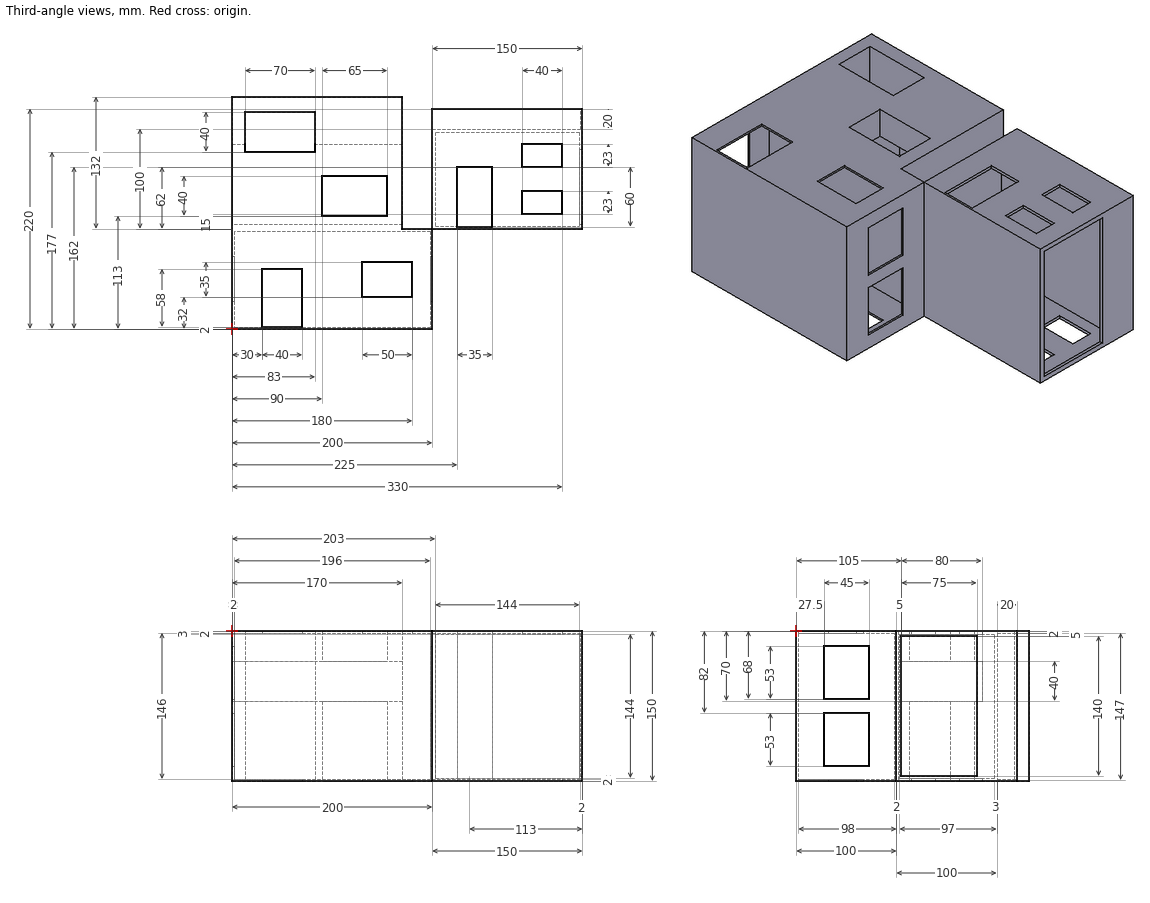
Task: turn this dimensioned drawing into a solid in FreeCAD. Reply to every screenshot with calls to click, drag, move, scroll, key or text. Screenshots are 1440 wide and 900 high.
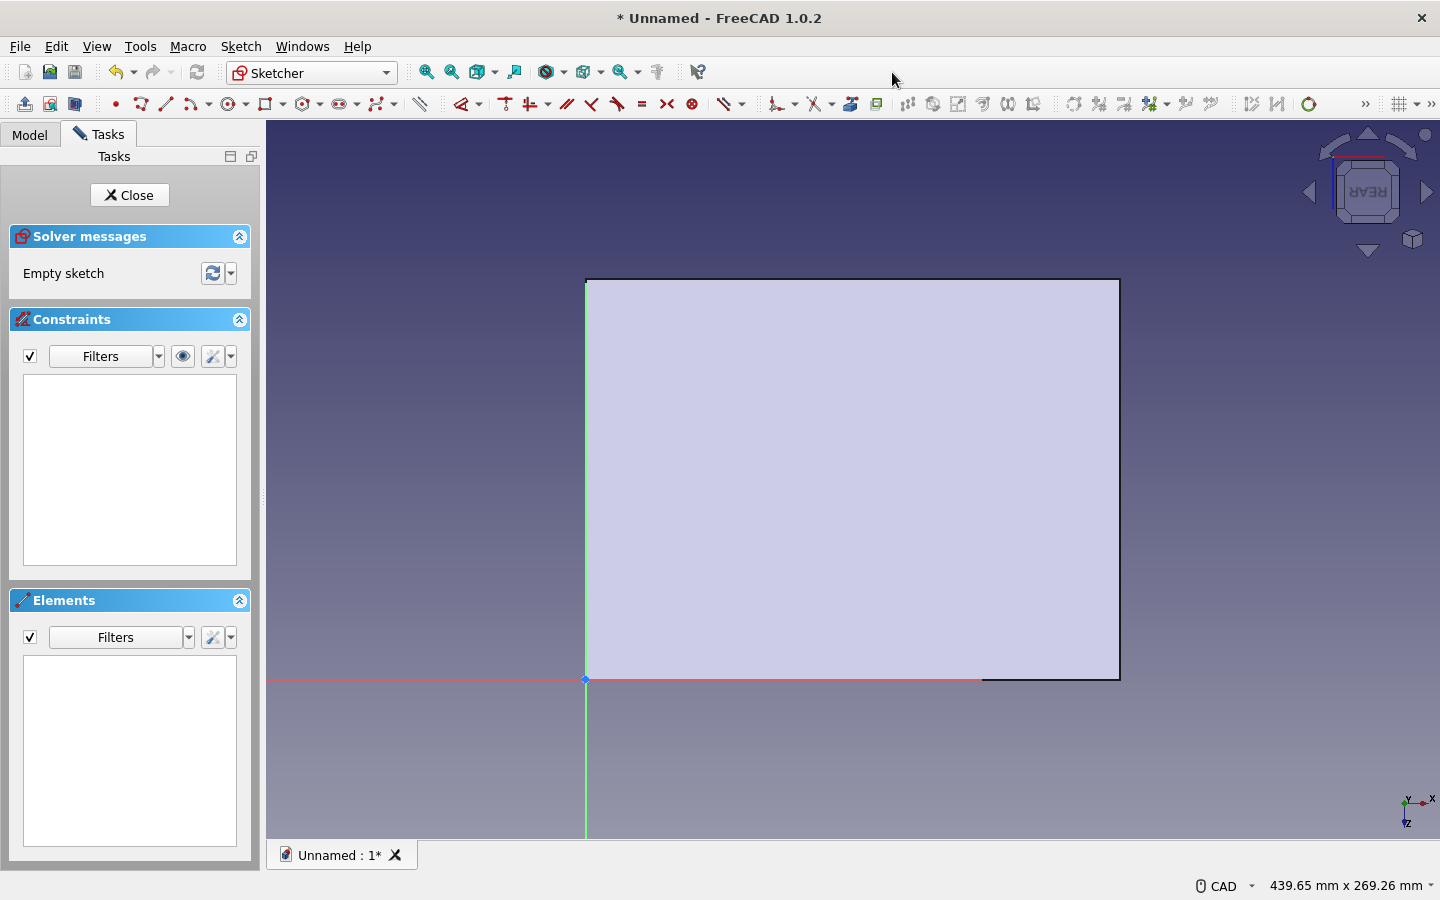
click(264, 104)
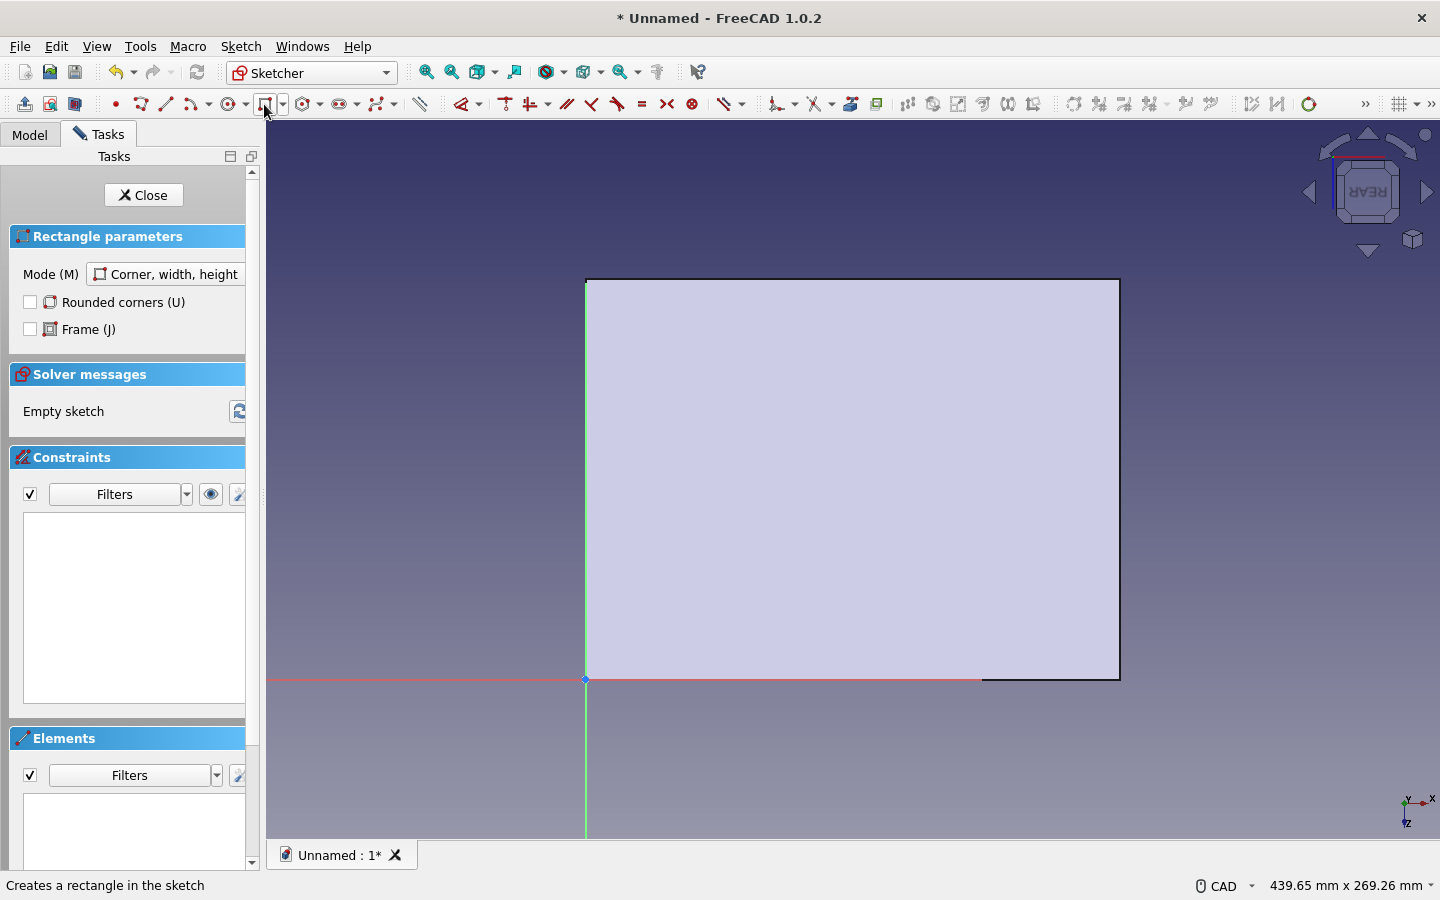
scroll(591, 285, up, 6)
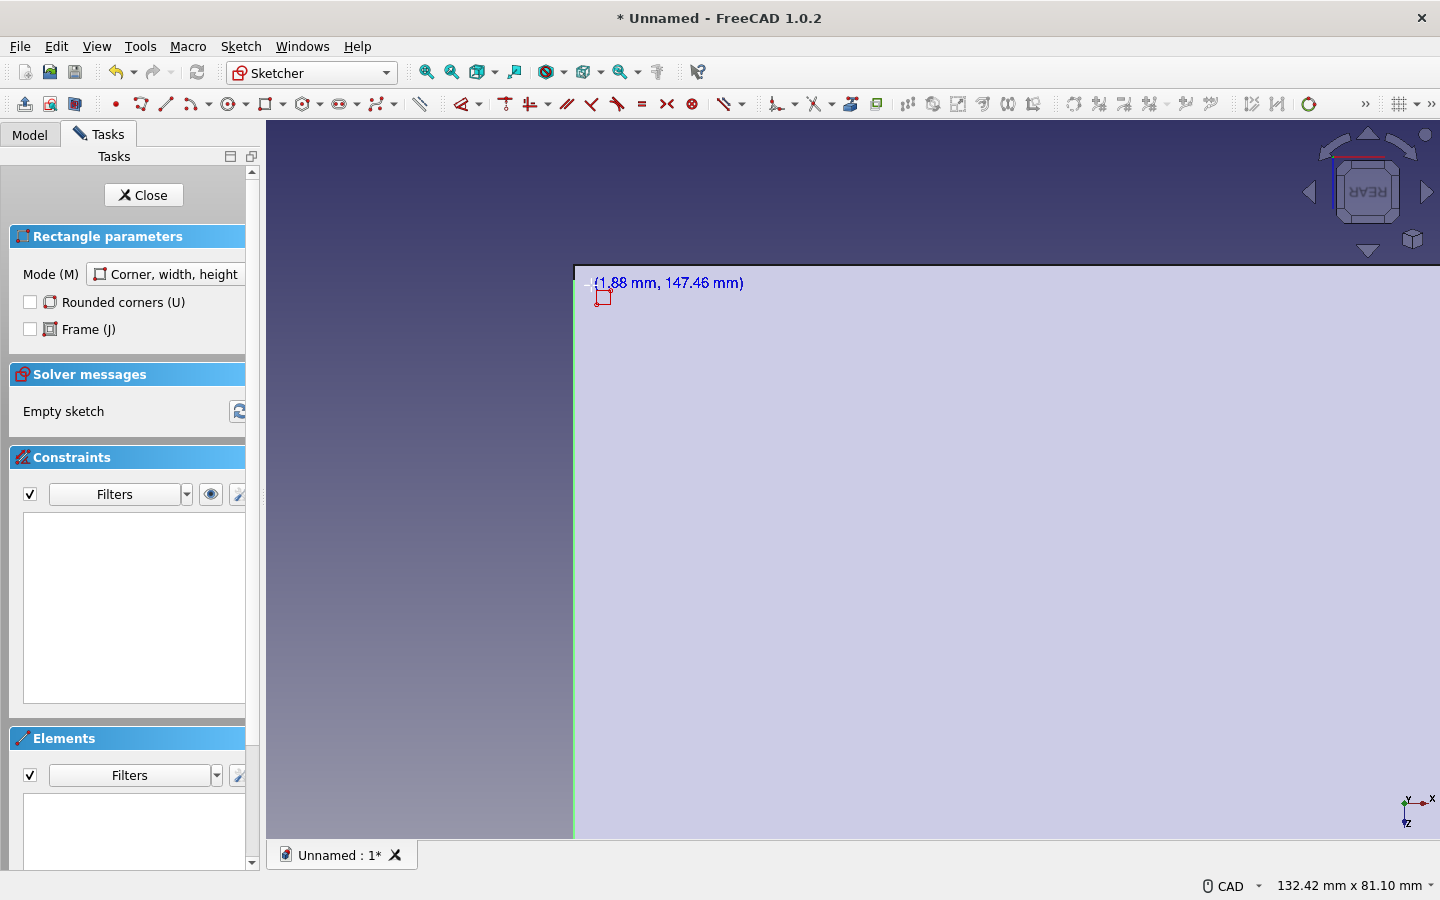
click(591, 283)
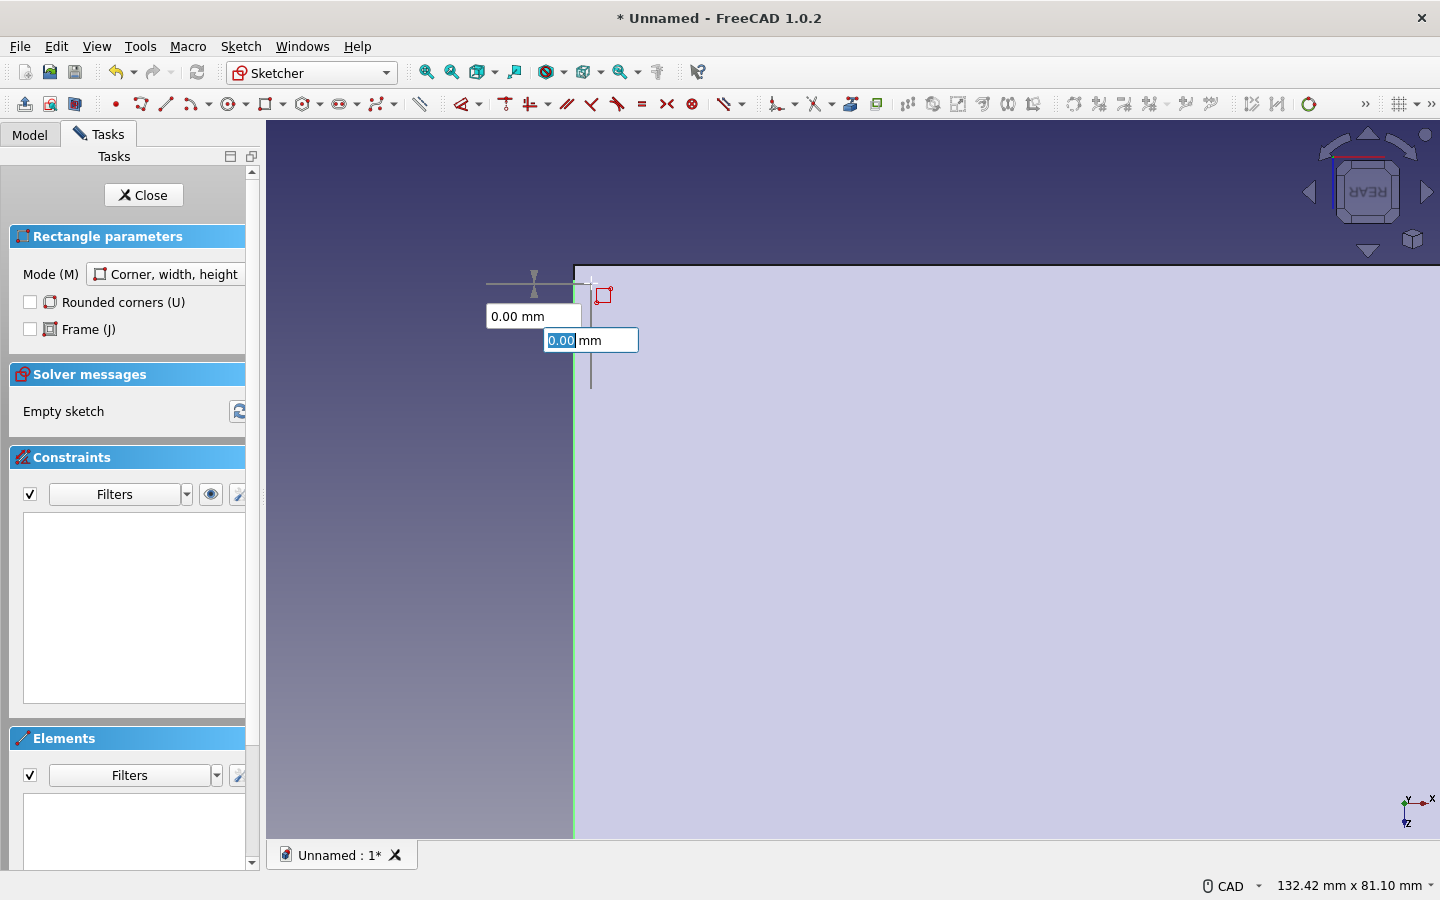
scroll(396, 212, down, 5)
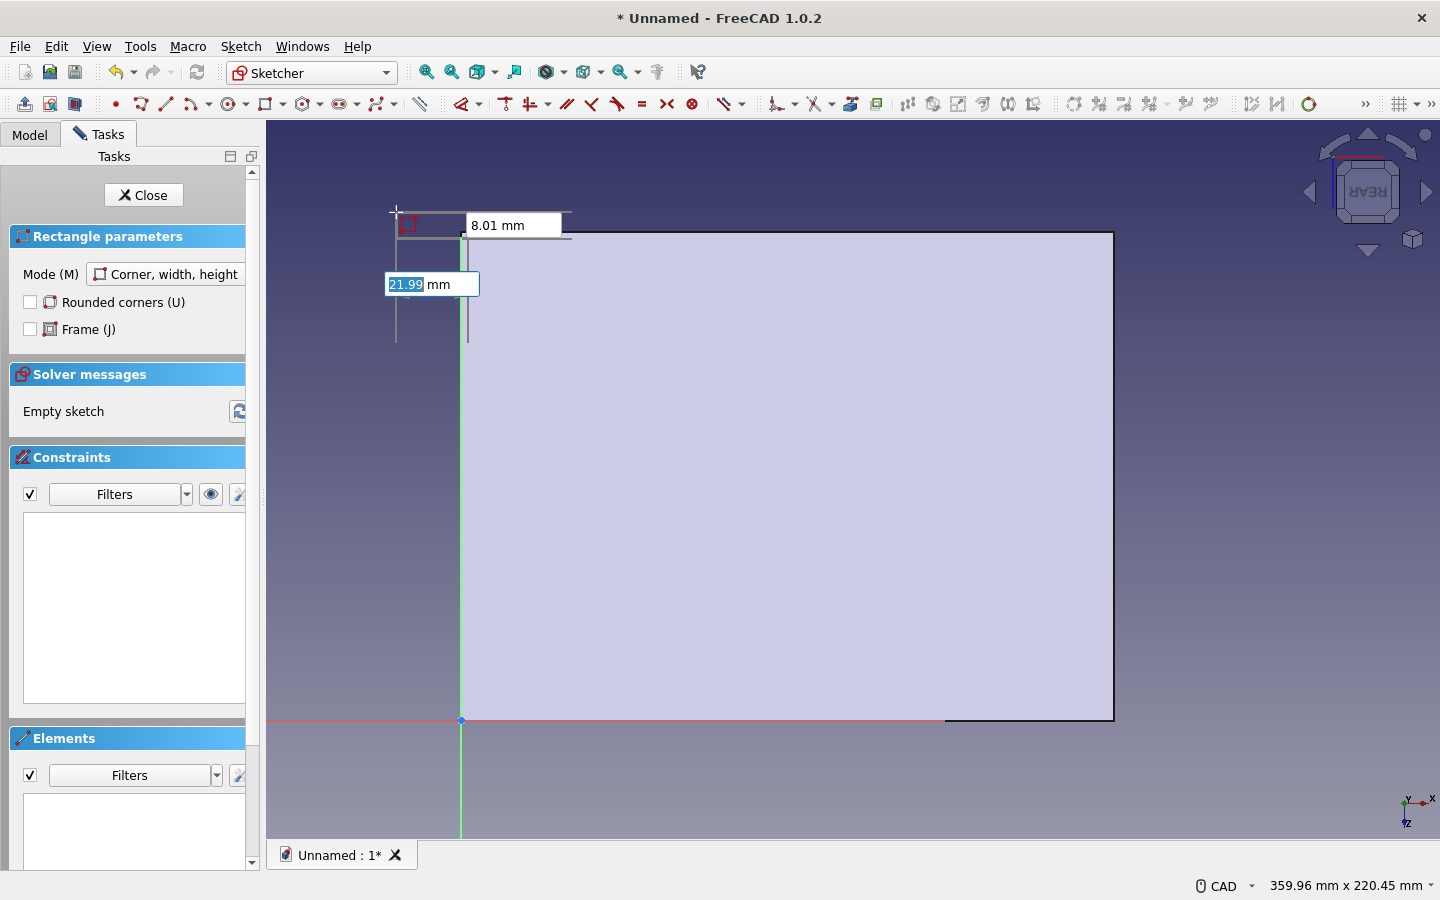
scroll(1107, 714, up, 5)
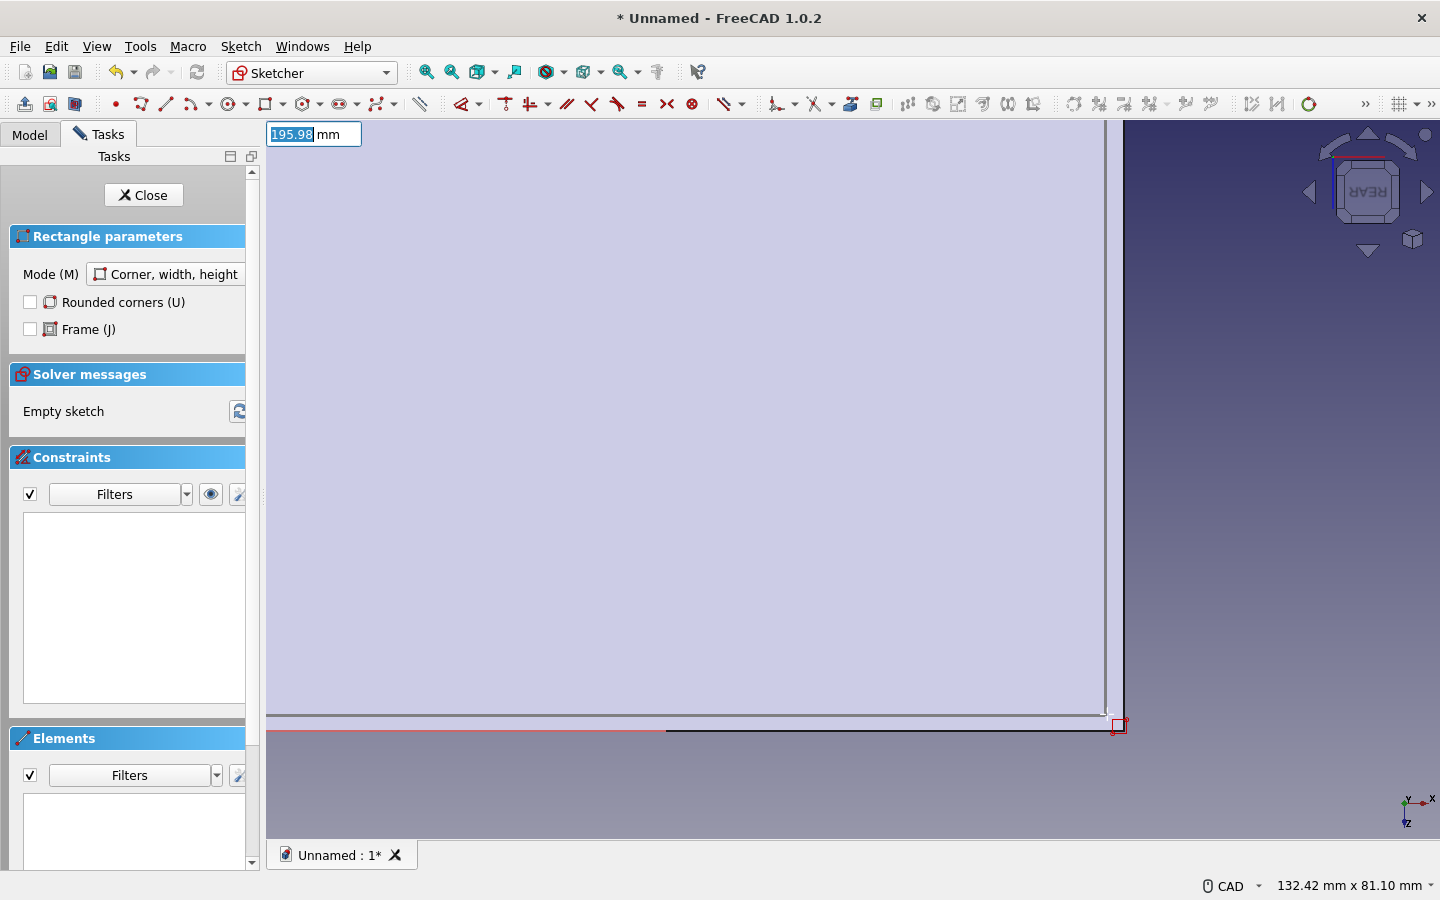
click(1106, 714)
key(Escape)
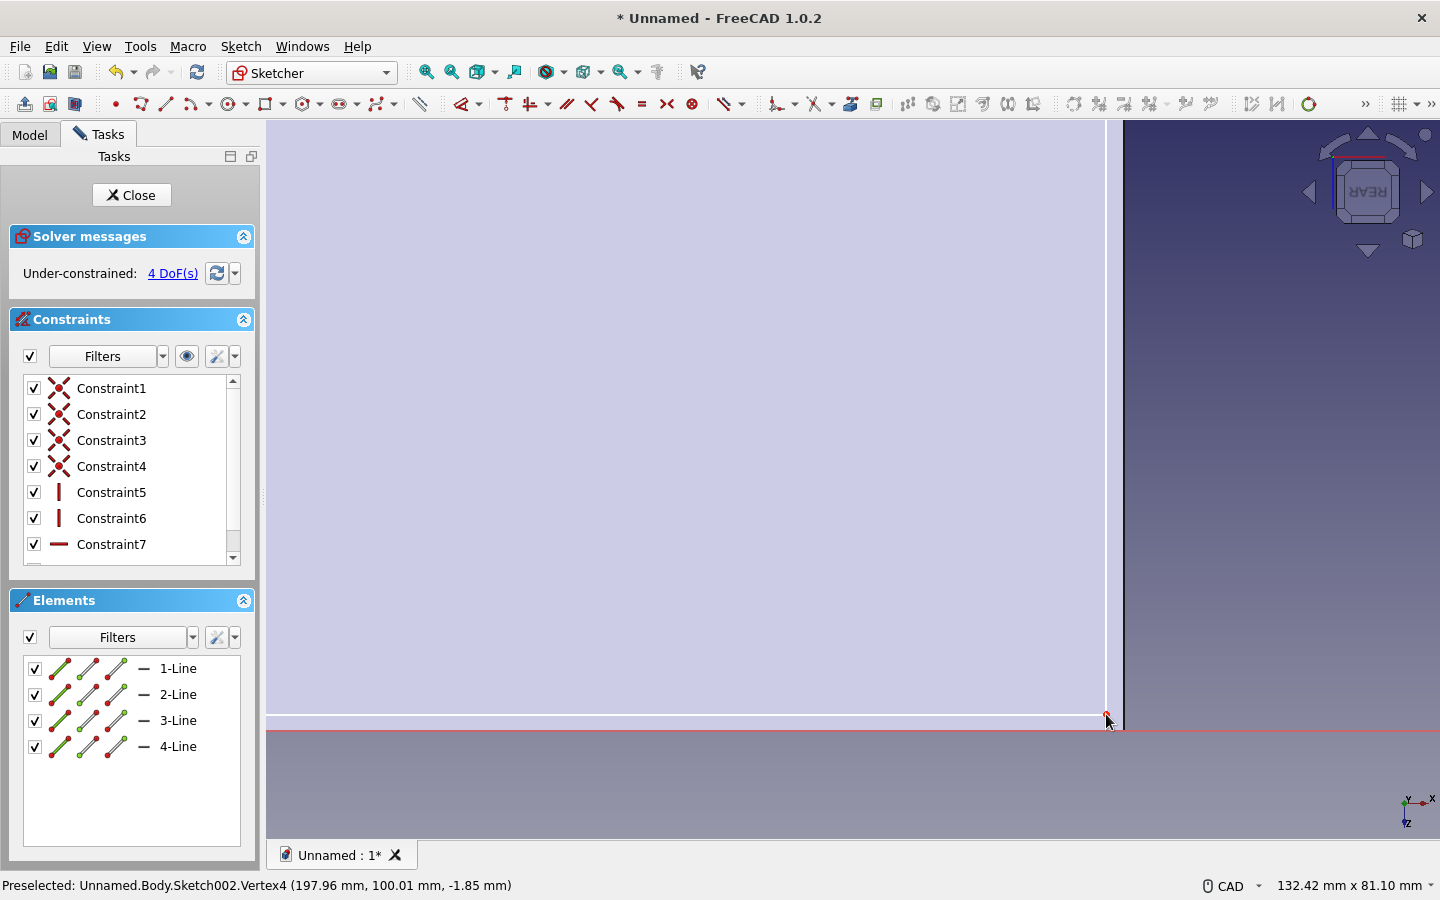
click(460, 104)